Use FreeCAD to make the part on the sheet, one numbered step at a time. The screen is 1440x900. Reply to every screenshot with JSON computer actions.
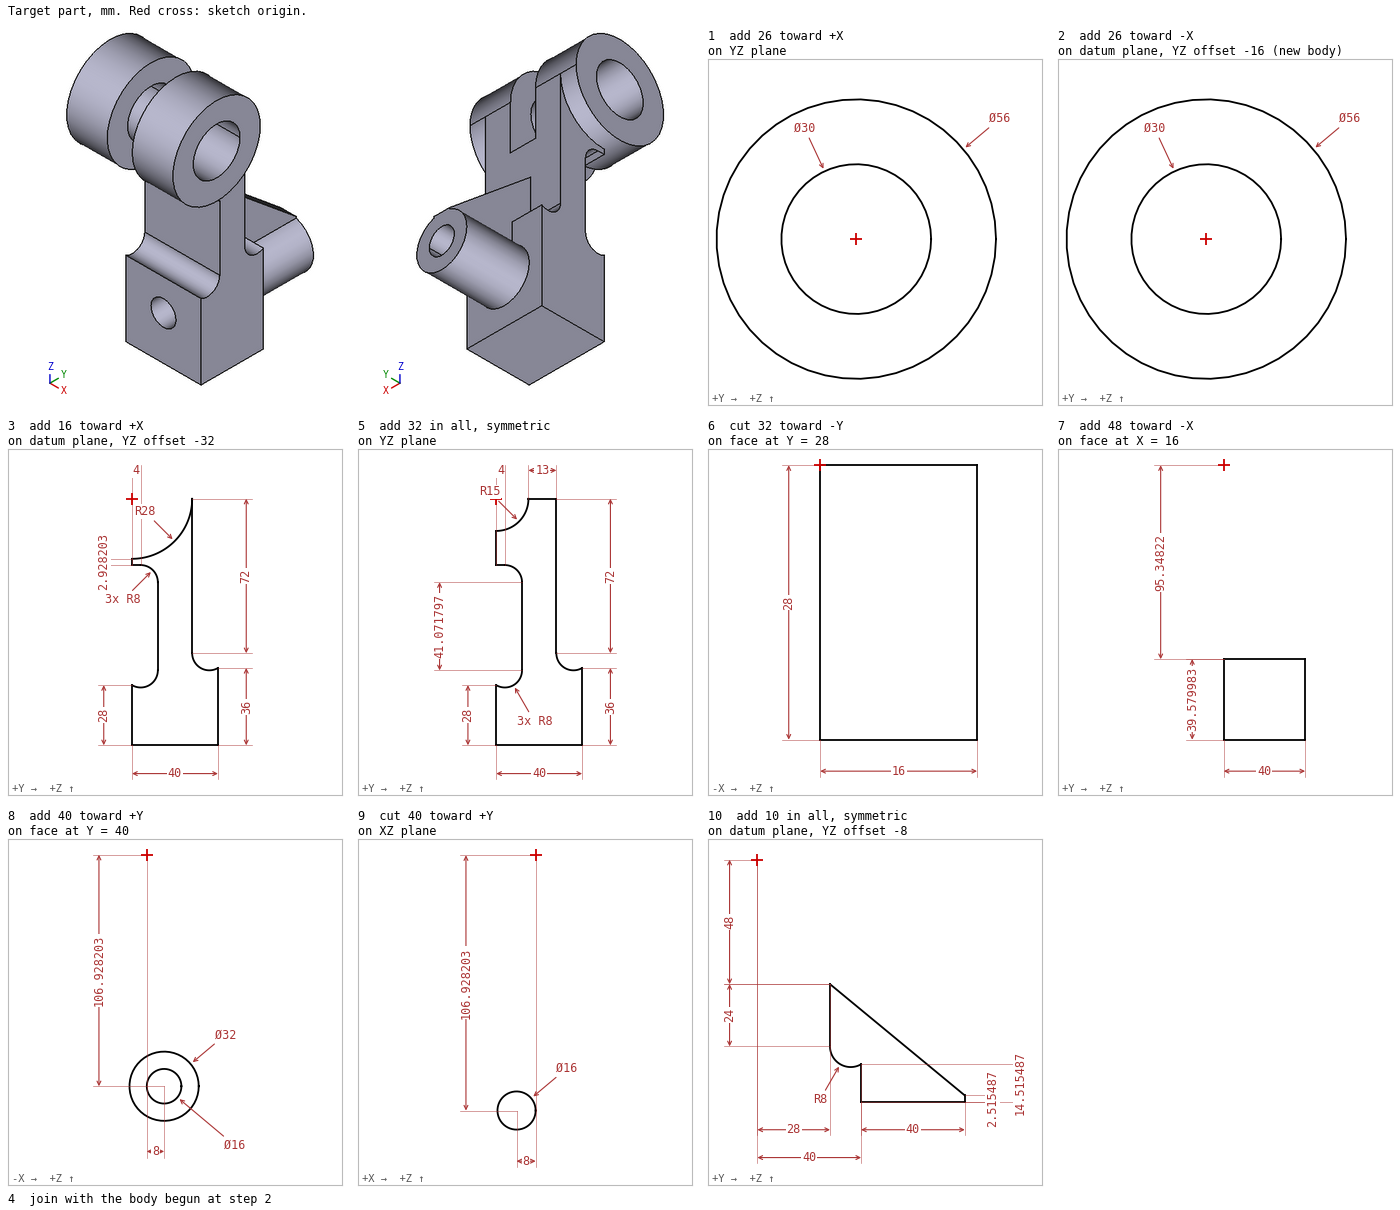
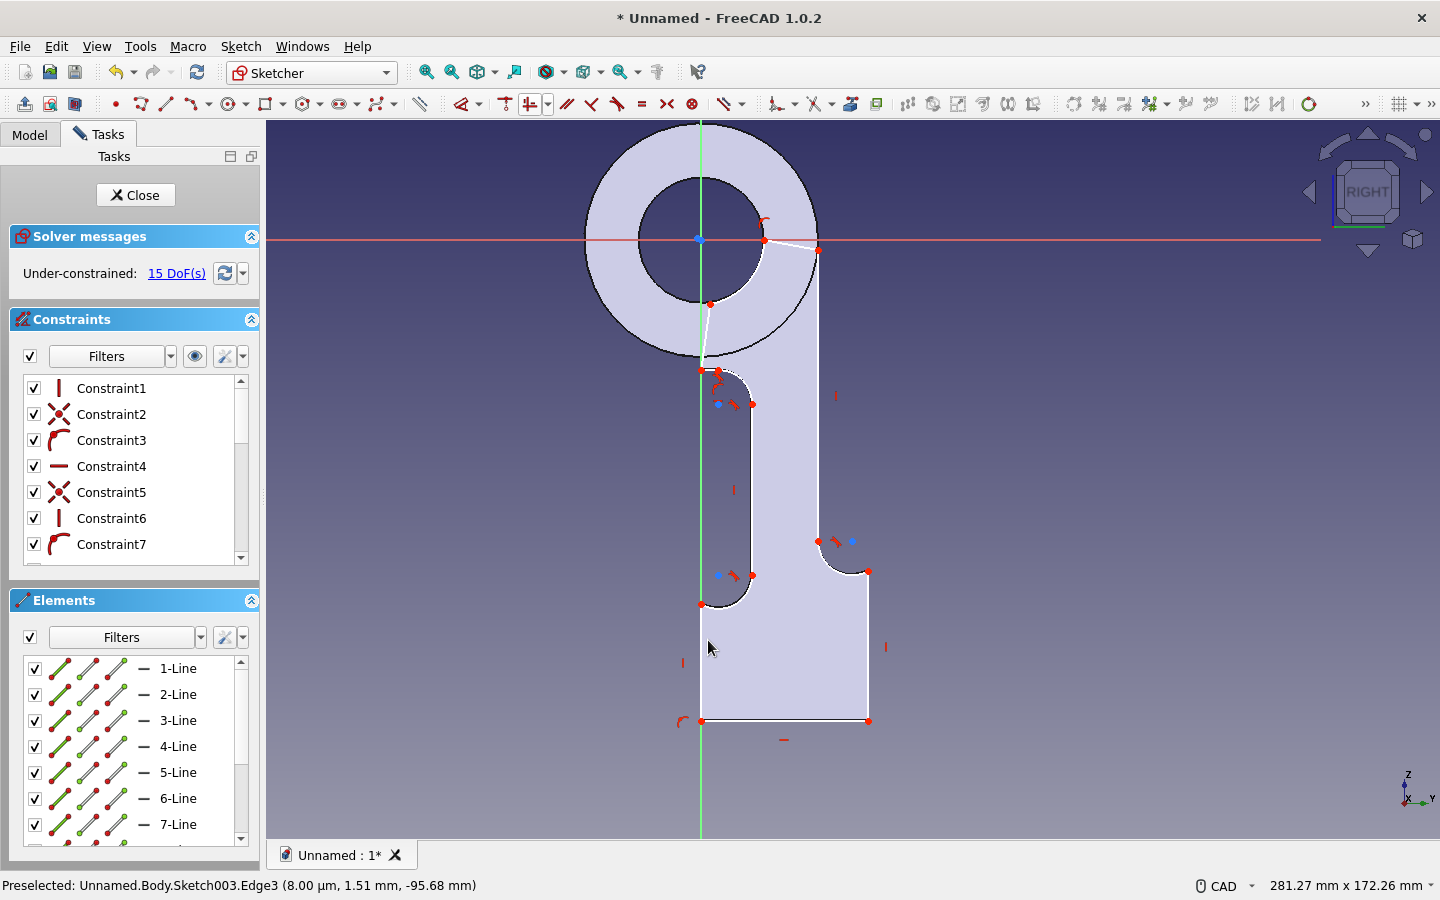
{"action": "scroll", "coordinate": [708, 324], "scroll_direction": "up", "scroll_amount": 4}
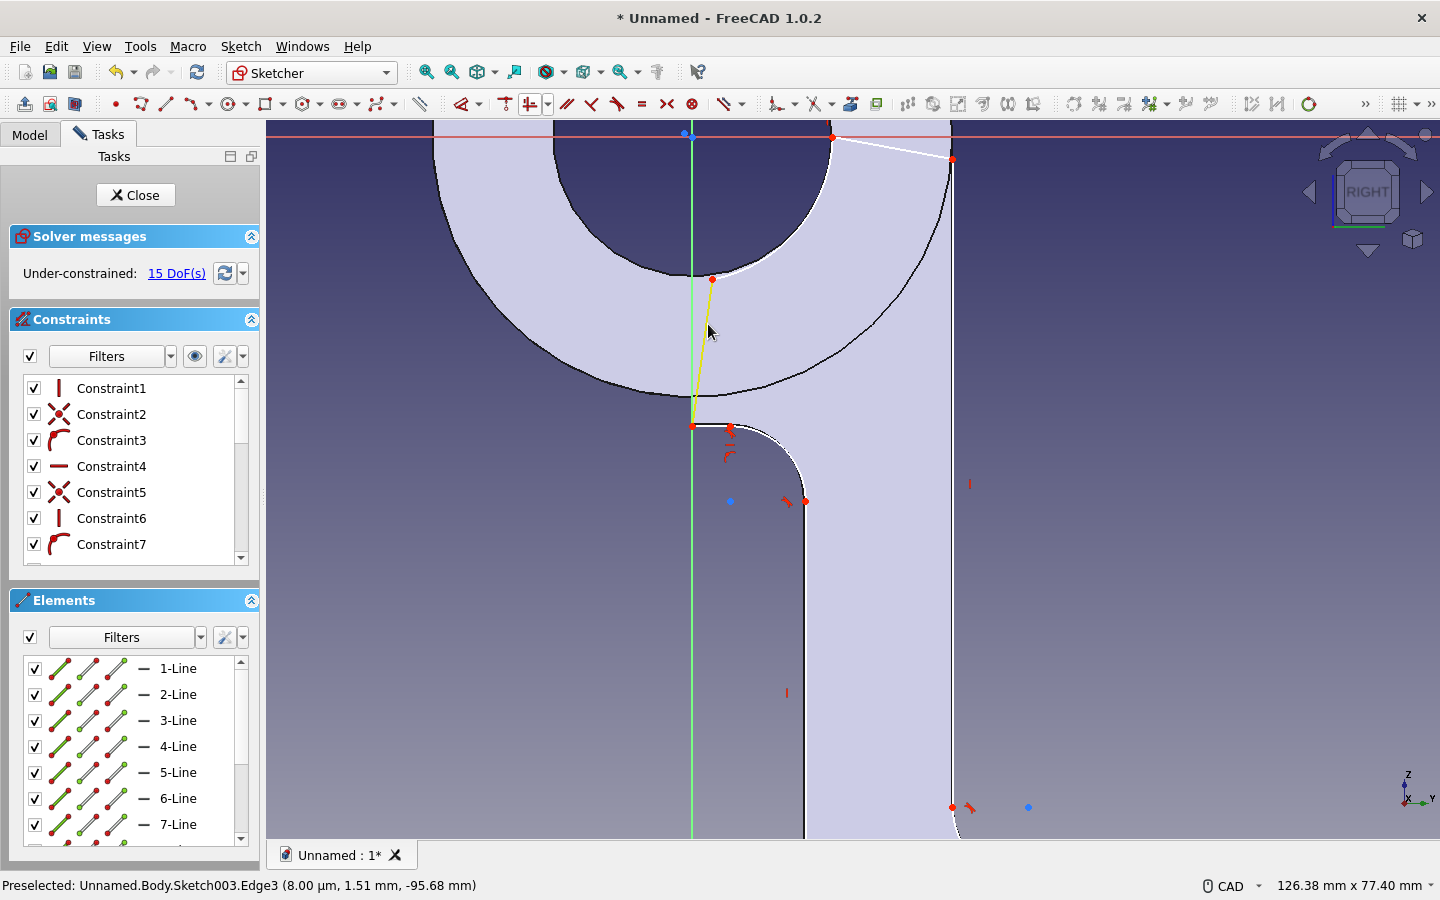
{"action": "left_click", "coordinate": [706, 323]}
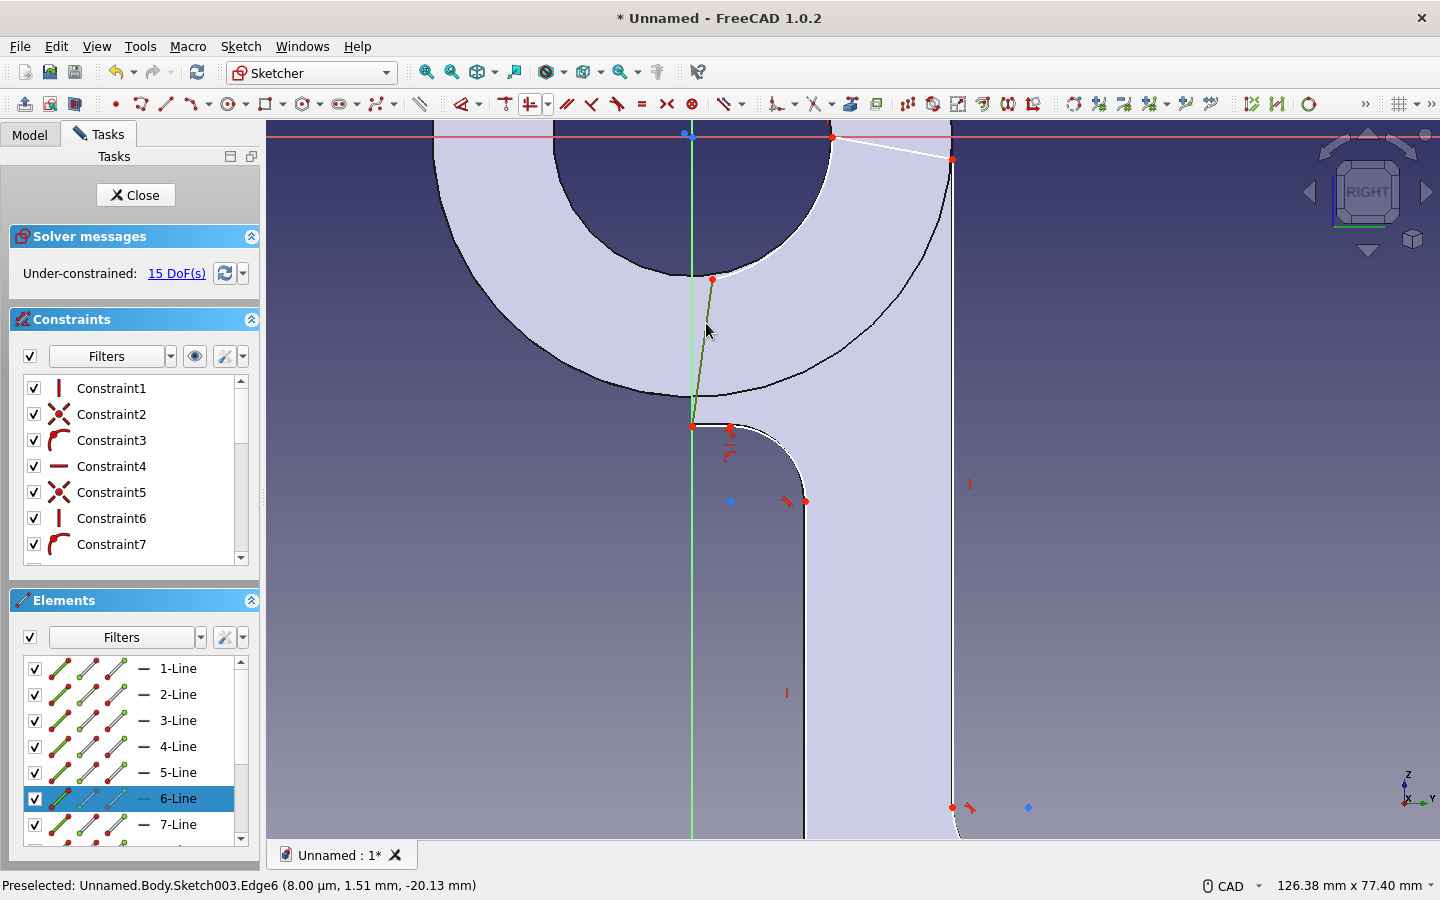
{"action": "key", "text": "v"}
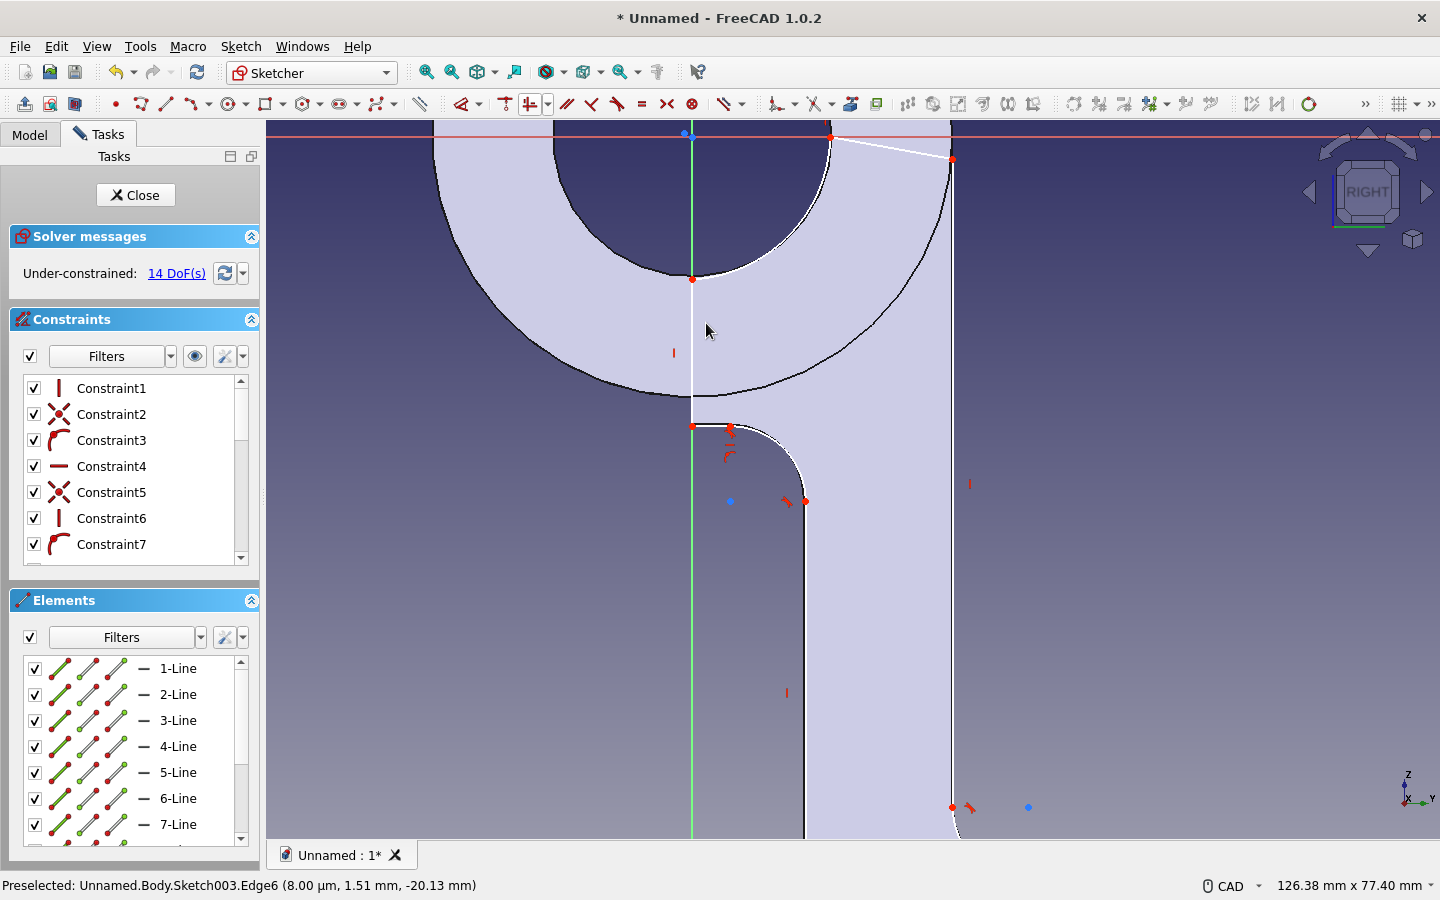
{"action": "left_click", "coordinate": [916, 153]}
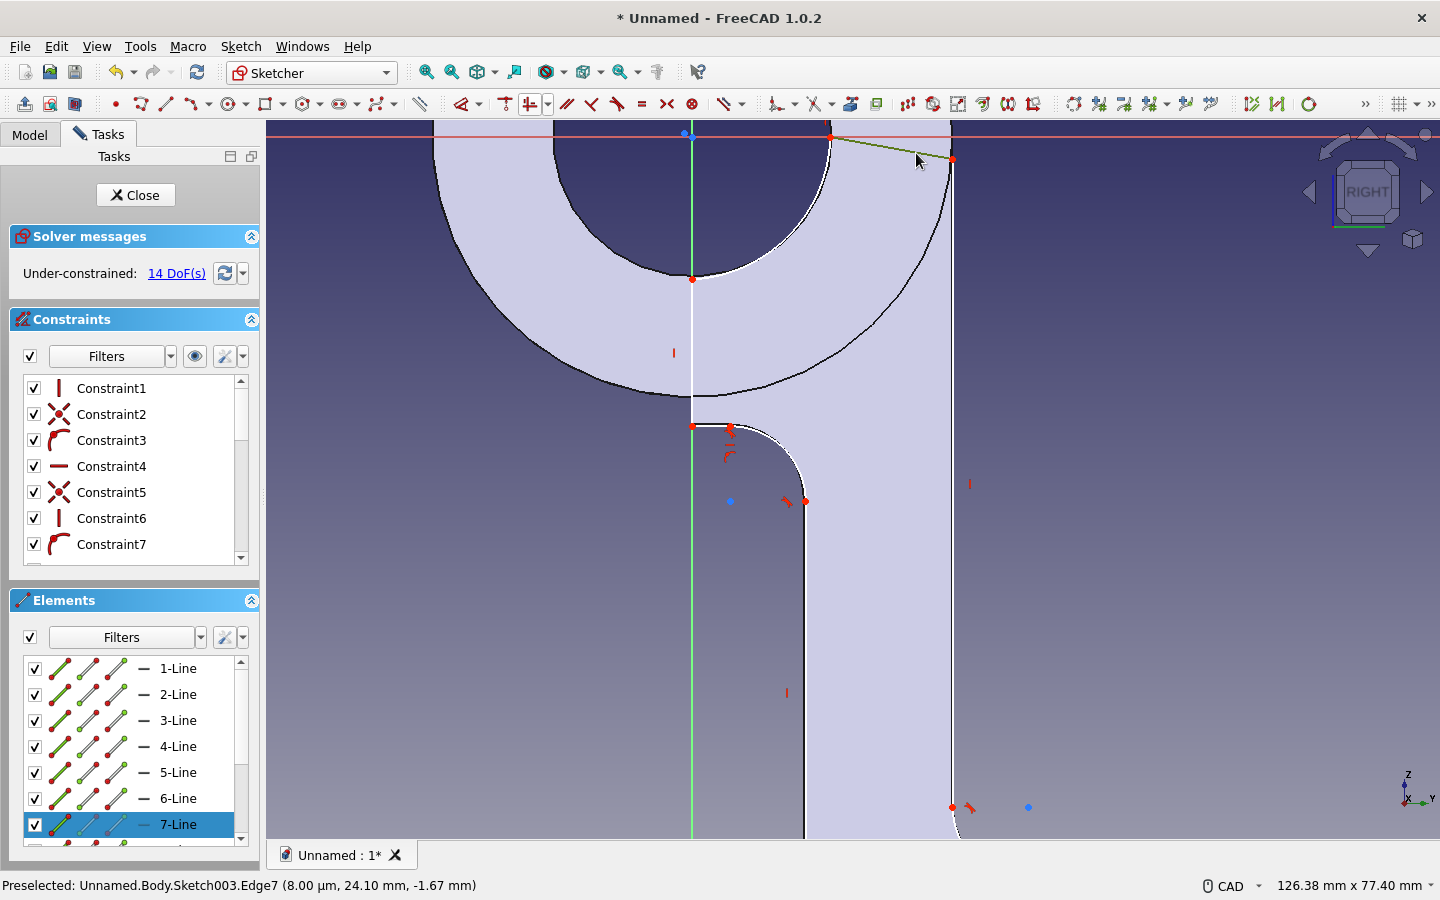
{"action": "key", "text": "h"}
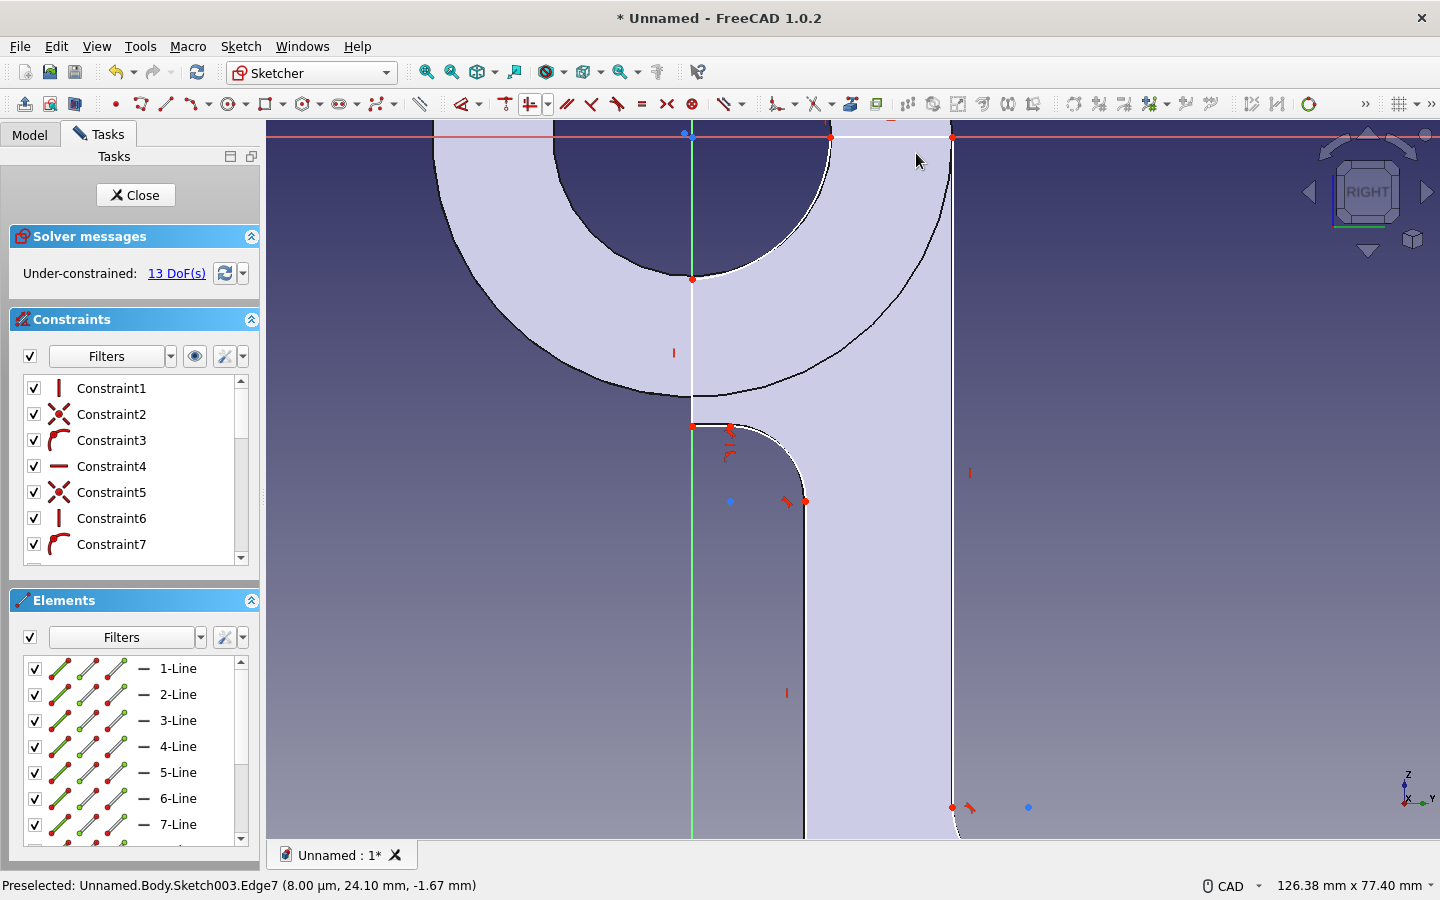
{"action": "scroll", "coordinate": [708, 323], "scroll_direction": "down", "scroll_amount": 4}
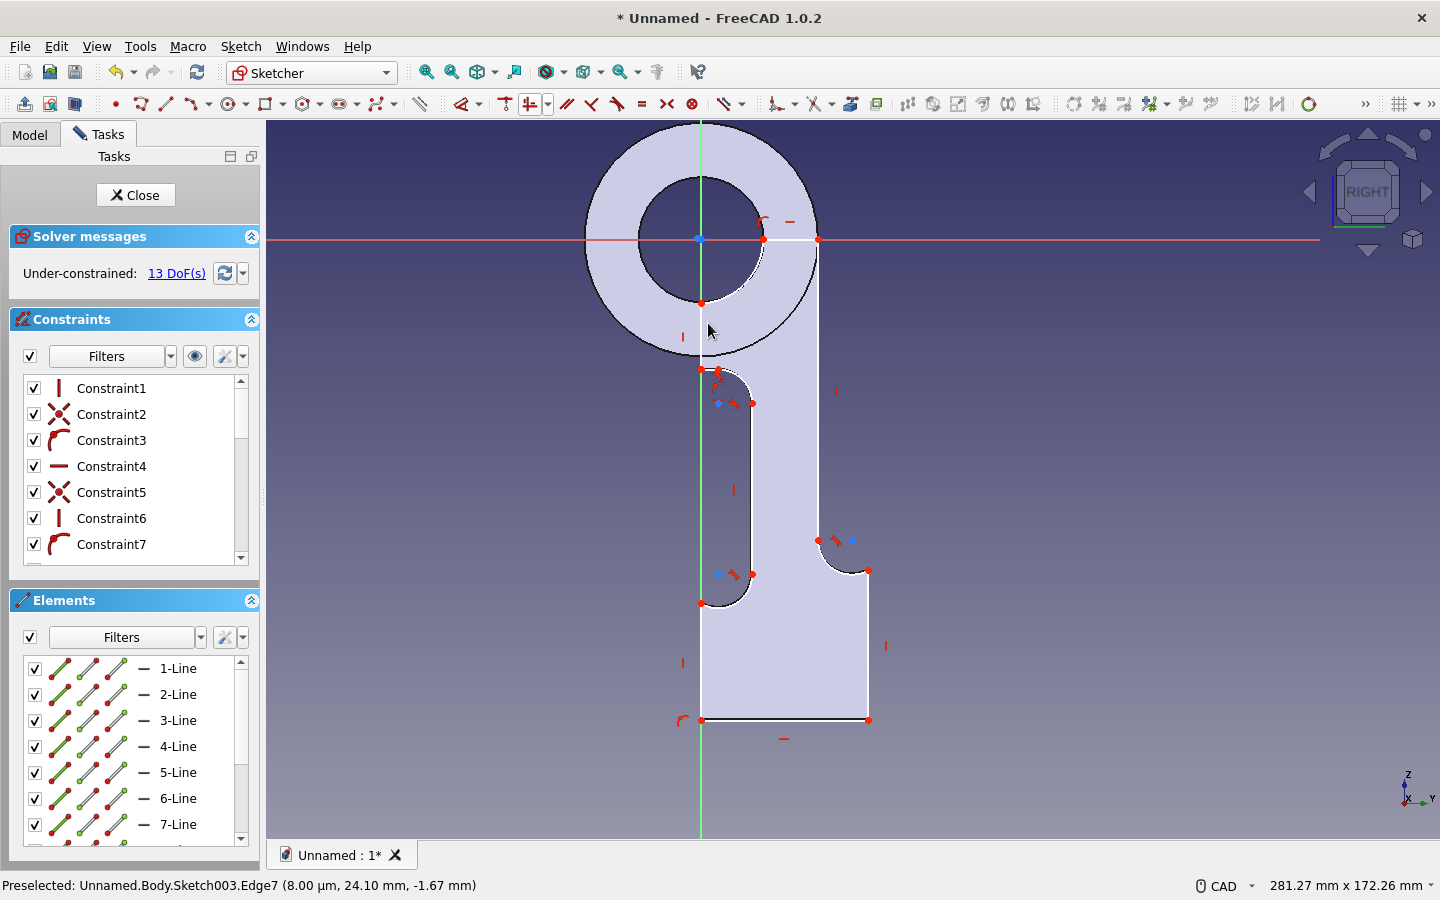
{"action": "left_click_drag", "start_coordinate": [688, 228], "coordinate": [711, 250]}